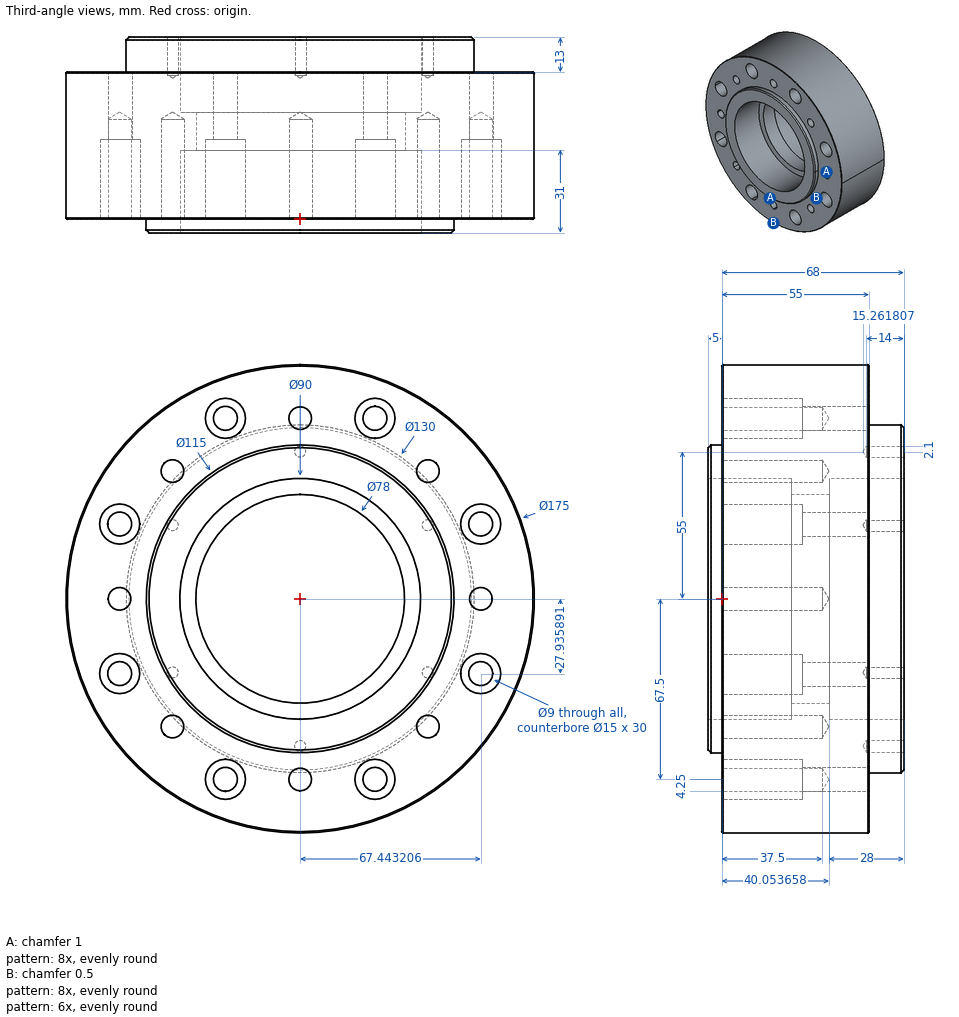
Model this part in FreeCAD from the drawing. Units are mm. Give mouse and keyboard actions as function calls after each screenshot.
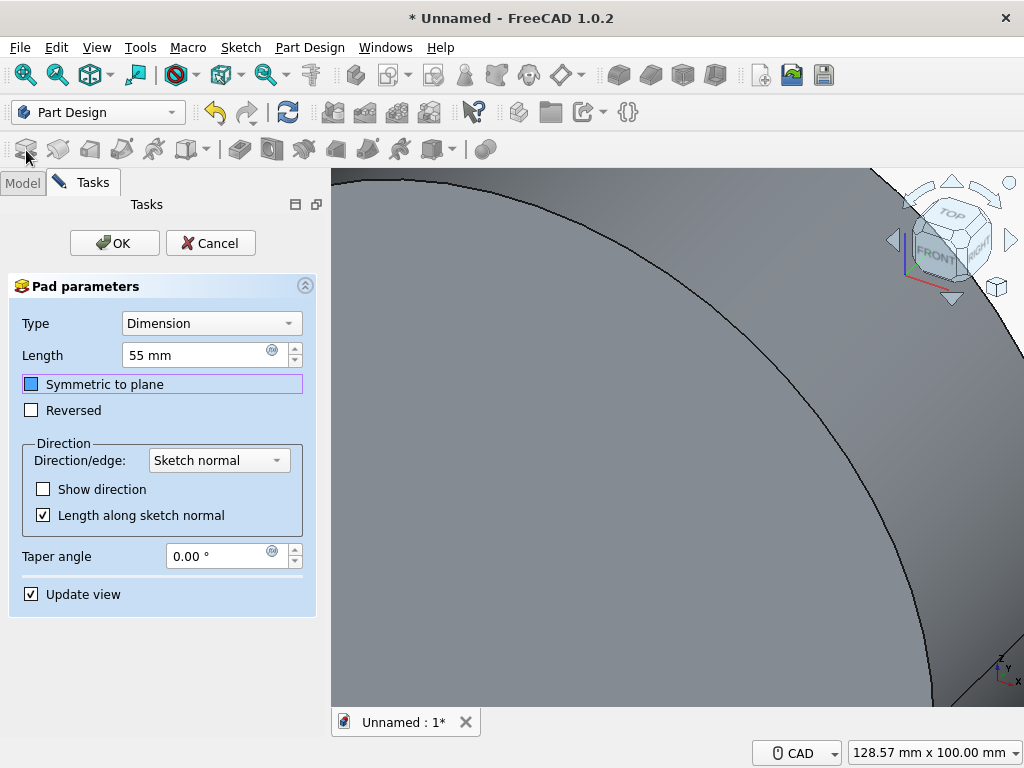
click(30, 410)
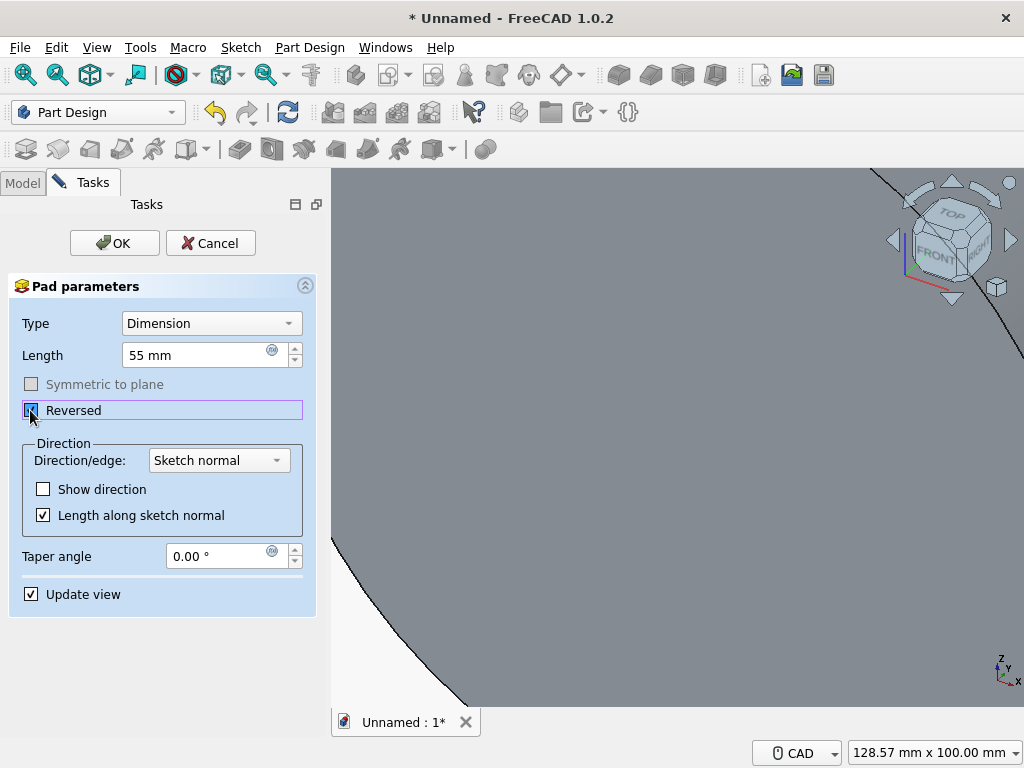
click(115, 243)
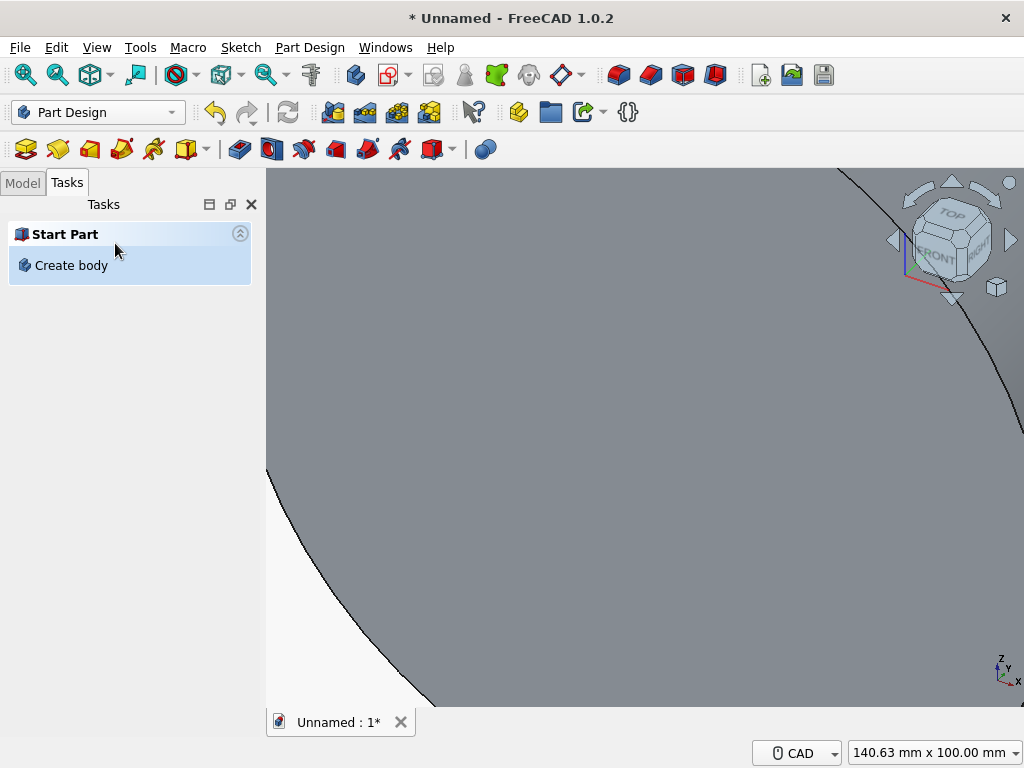
key(v)
key(f)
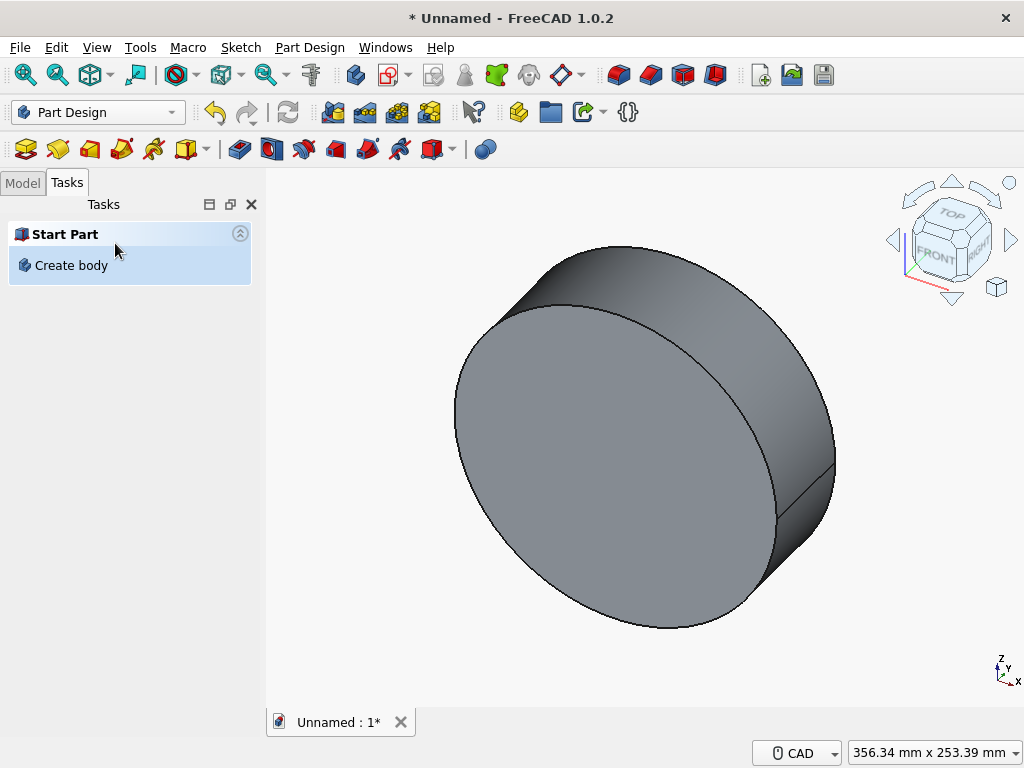
key(4)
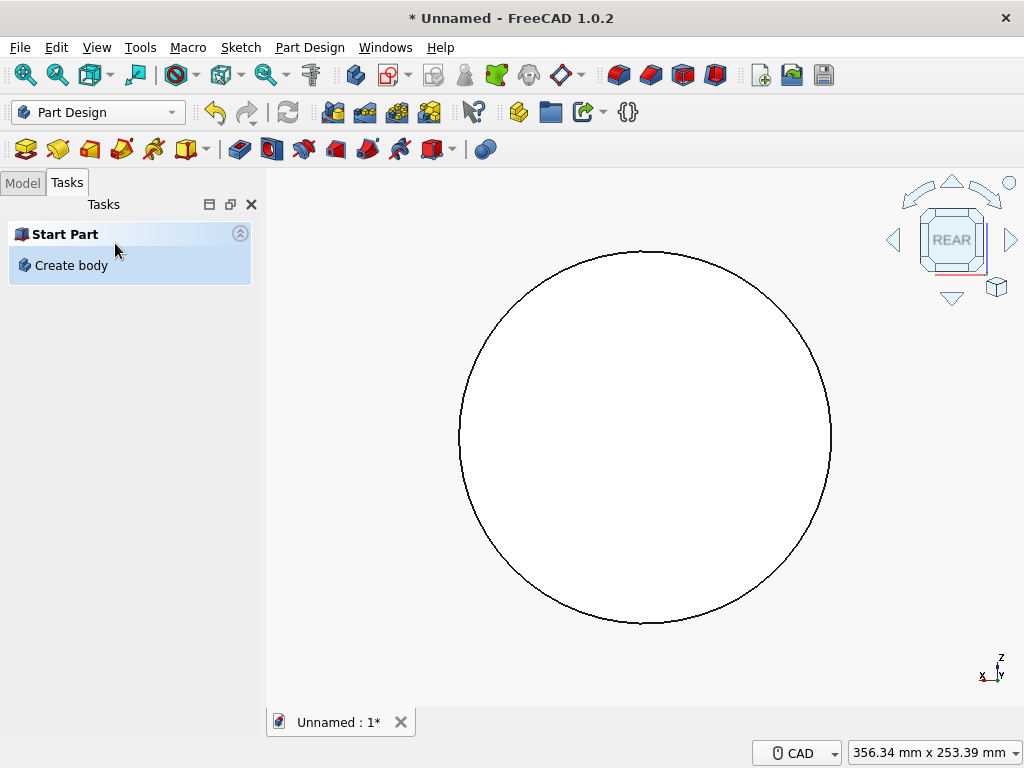
click(645, 437)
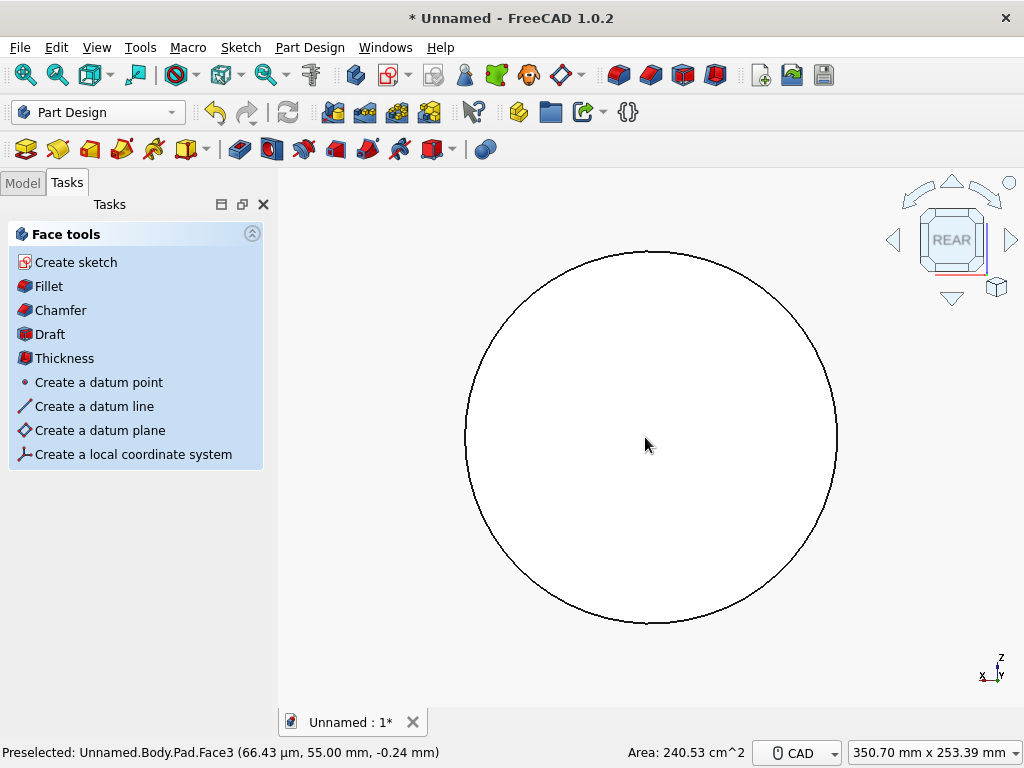
click(388, 76)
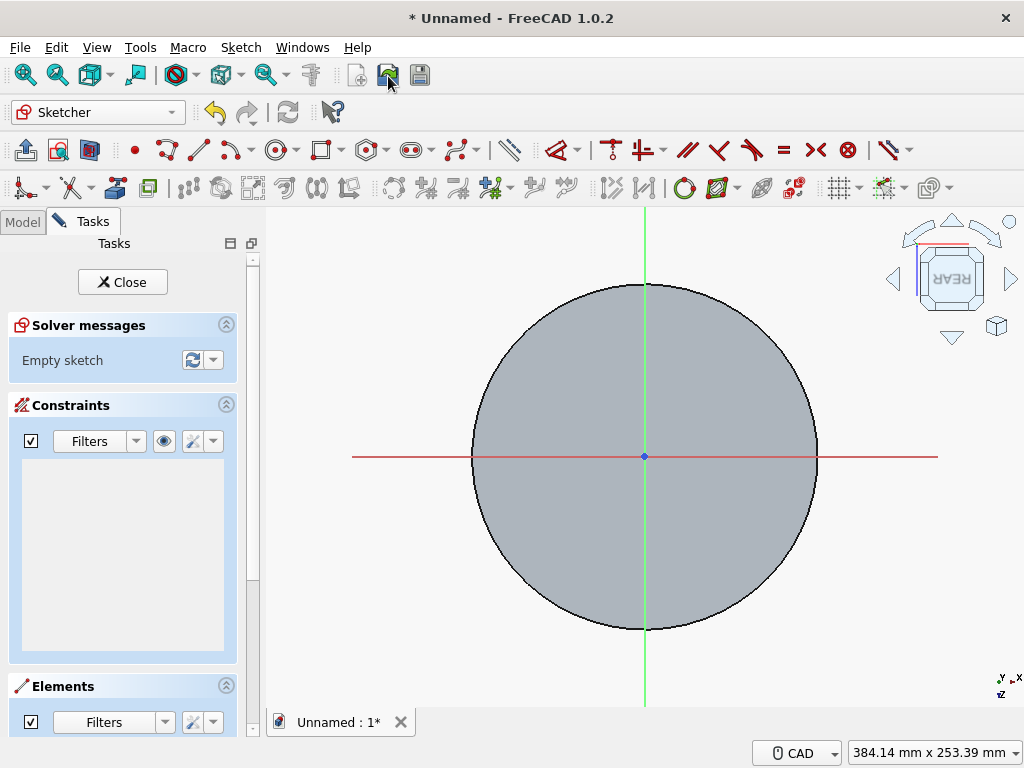
click(276, 150)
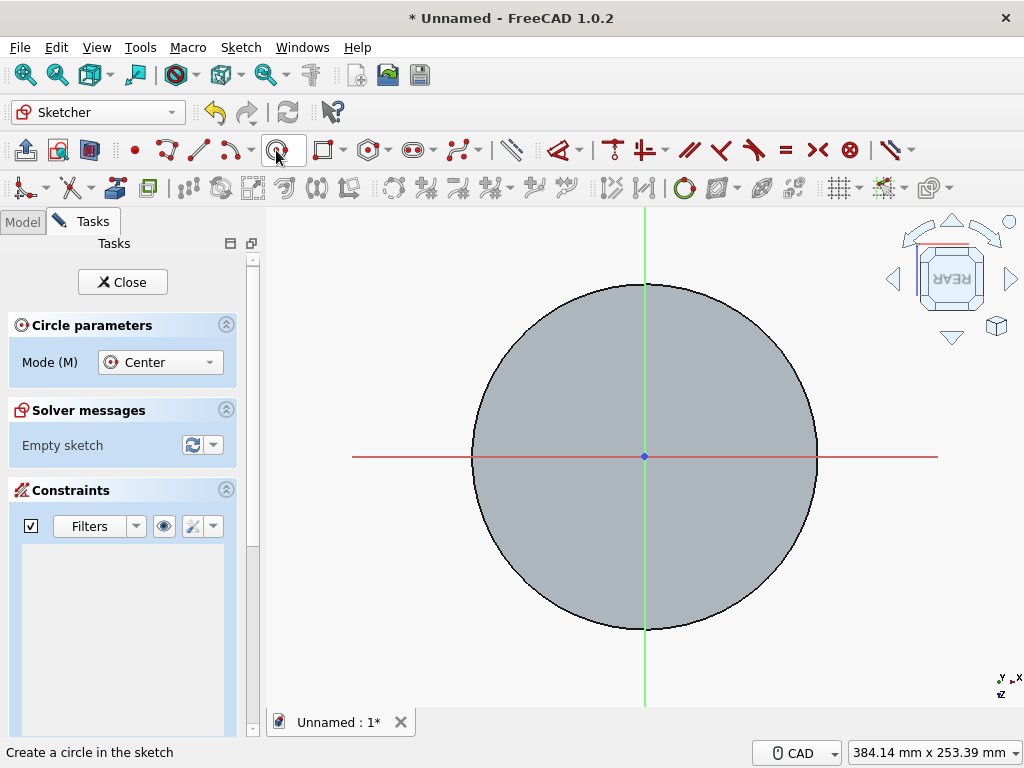
click(645, 457)
click(736, 366)
key(Escape)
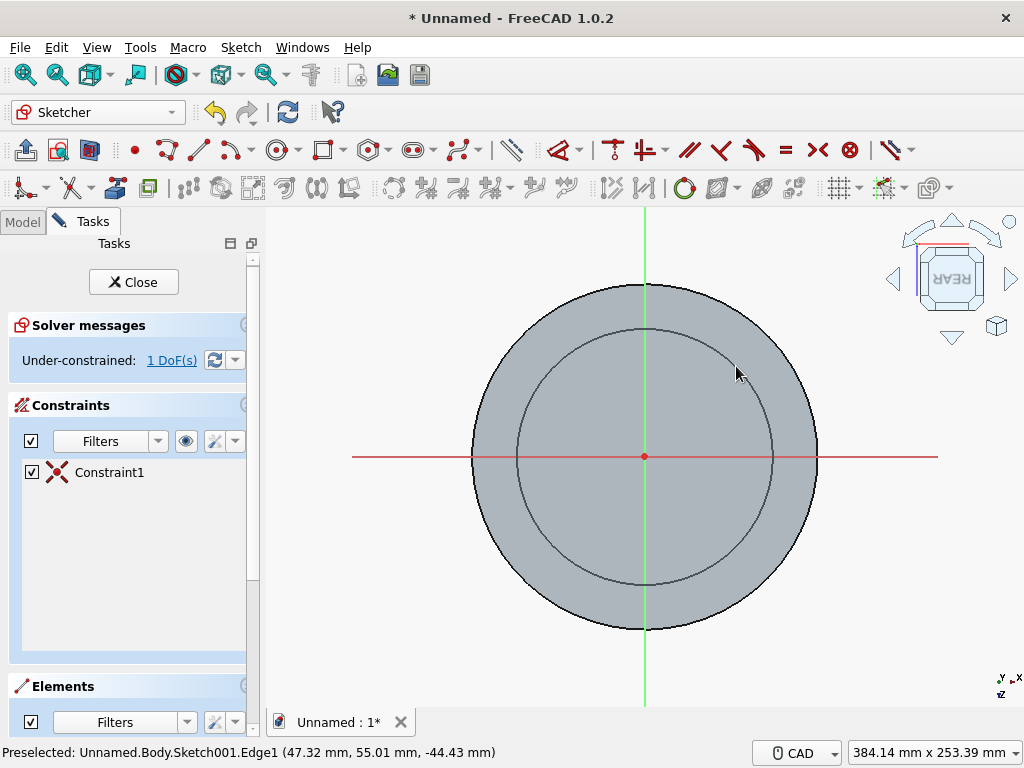
click(558, 150)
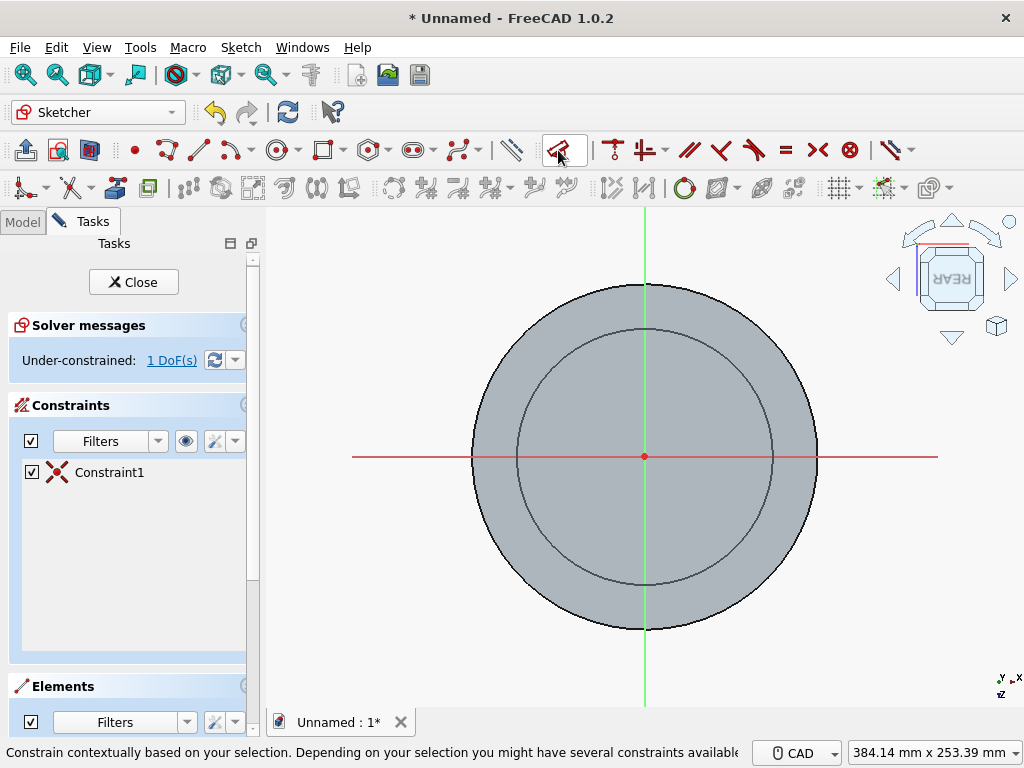
click(735, 366)
click(758, 343)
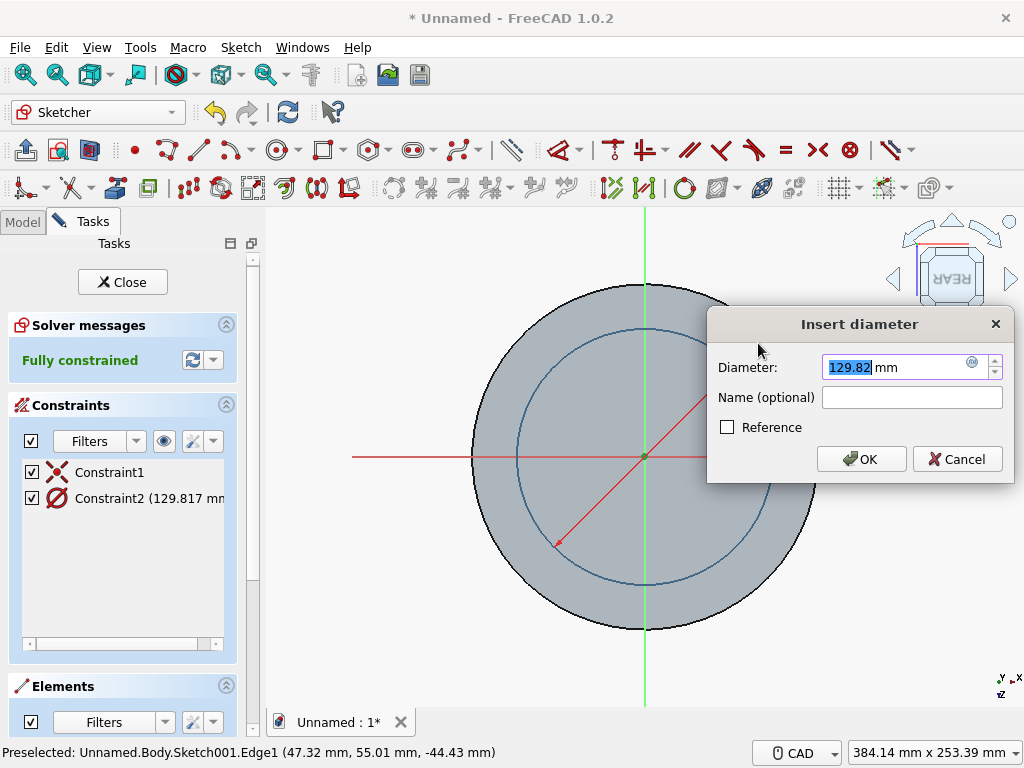
text(130)
key(Return)
key(Escape)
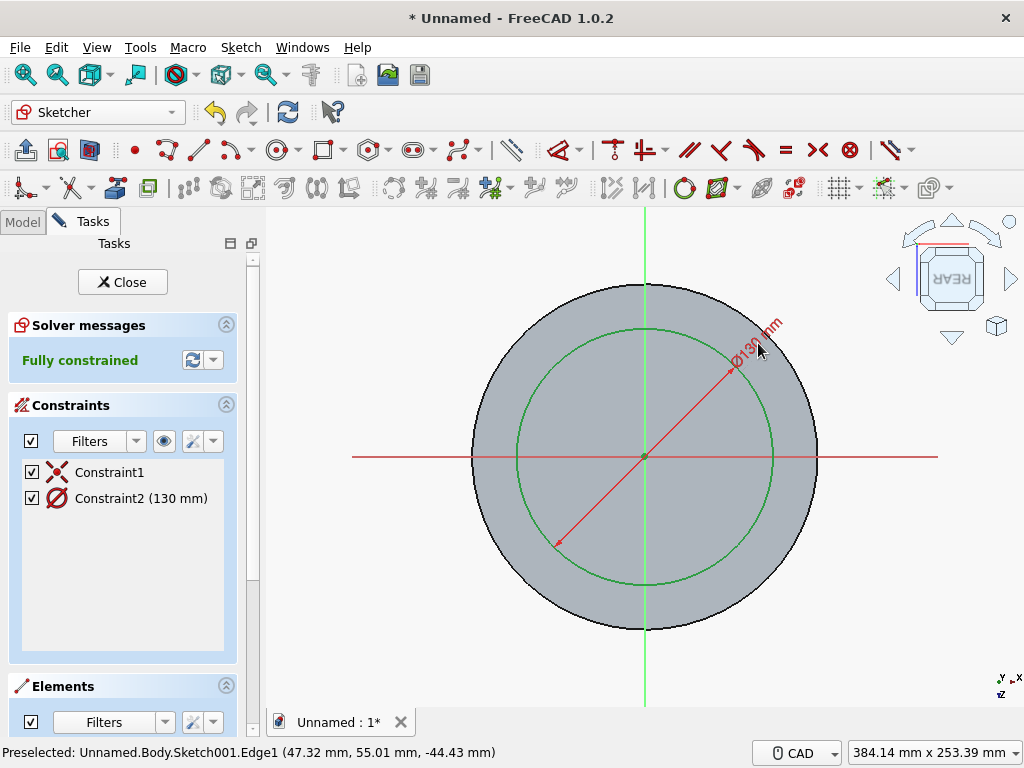
click(123, 282)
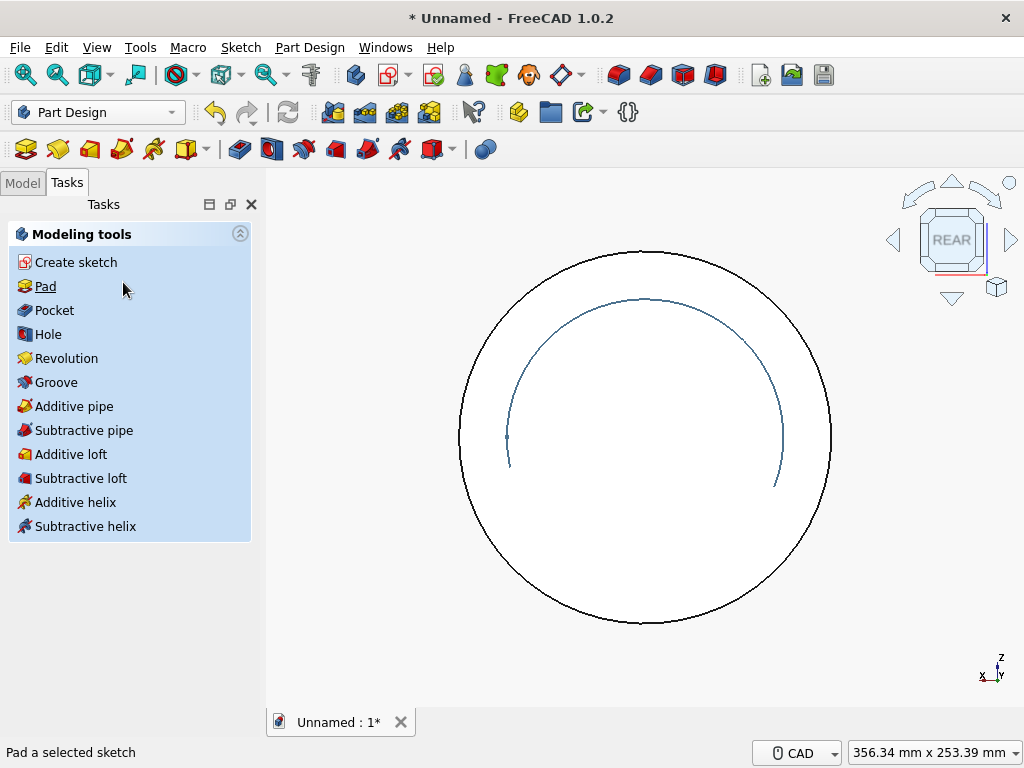
click(26, 150)